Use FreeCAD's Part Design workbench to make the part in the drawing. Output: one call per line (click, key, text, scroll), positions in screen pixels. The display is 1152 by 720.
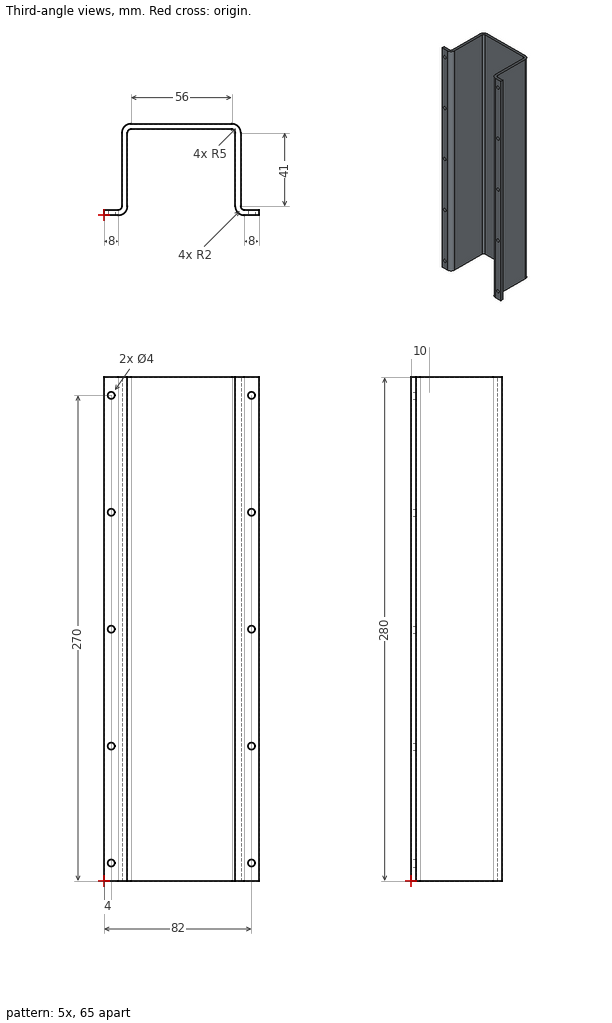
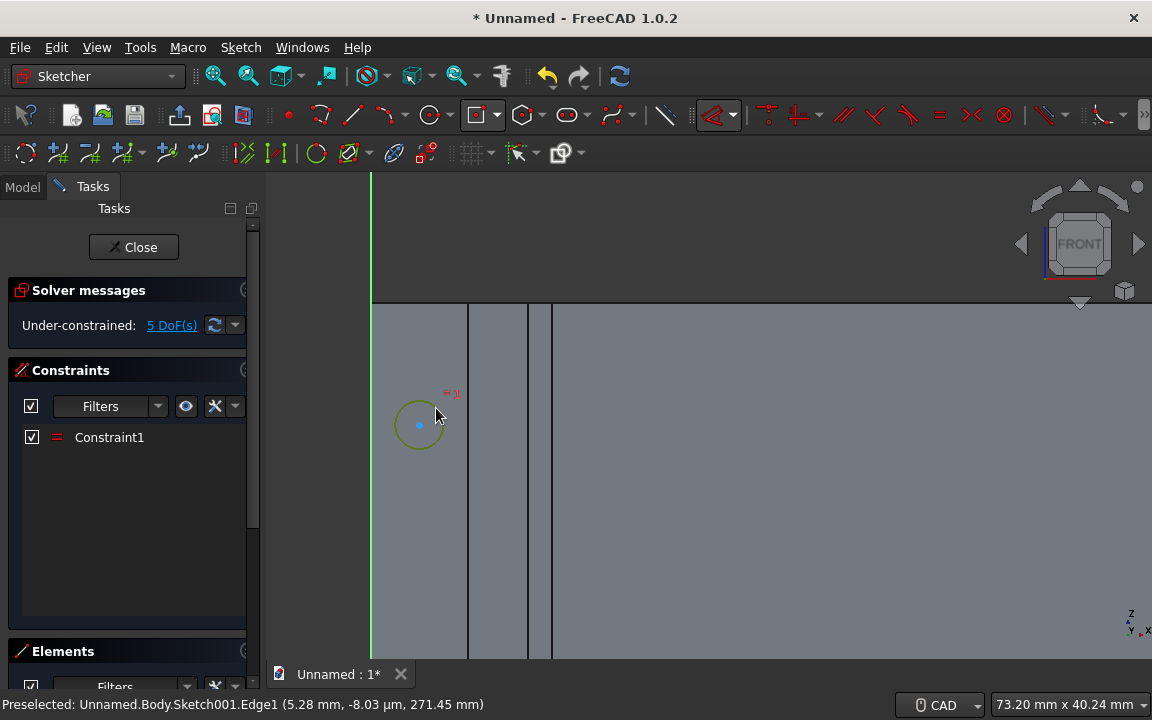
key(k)
key(o)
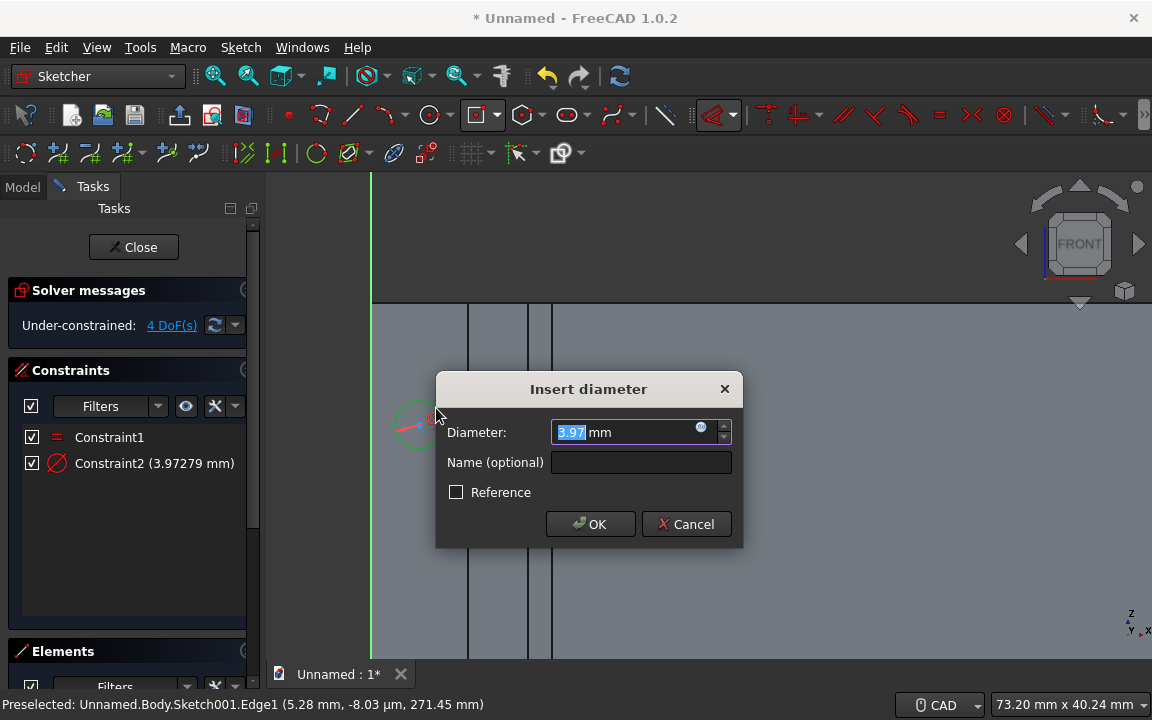
text(4)
key(Return)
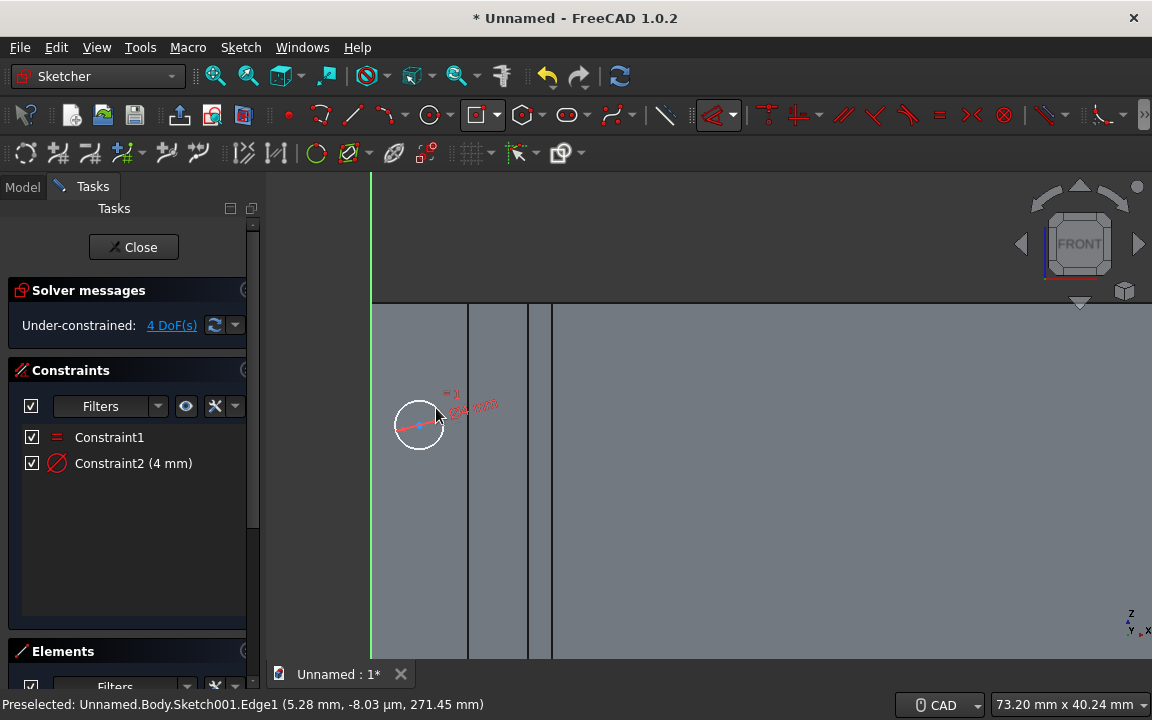
click(419, 425)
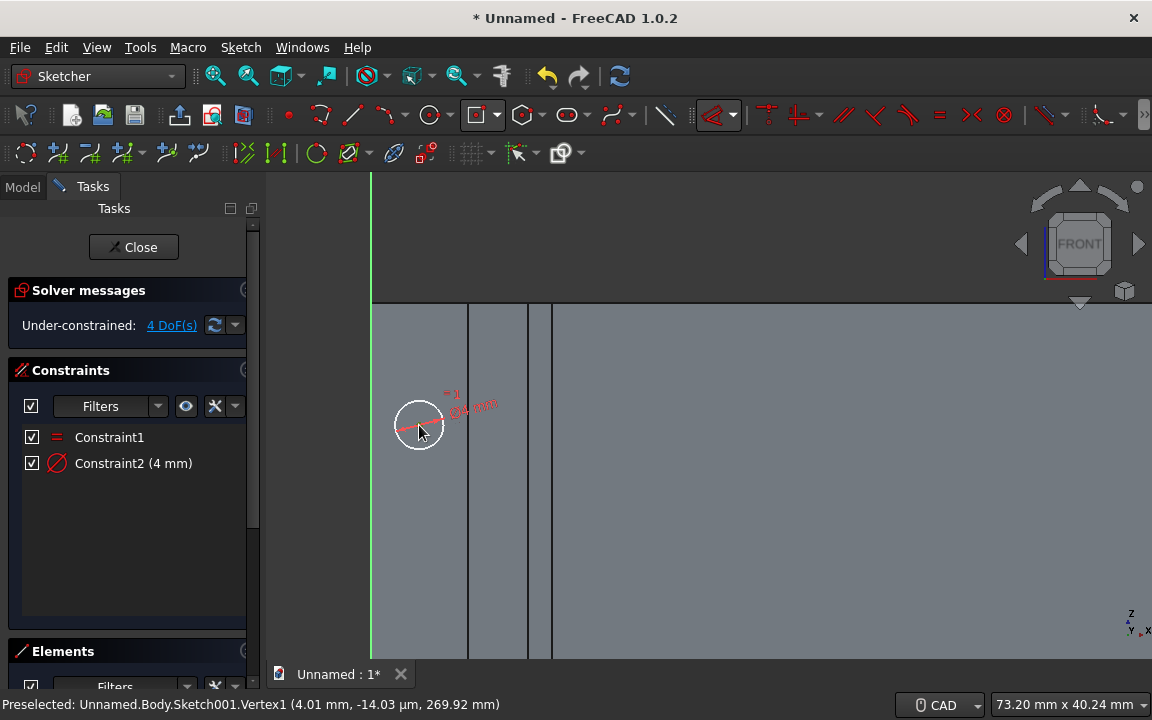
key(l)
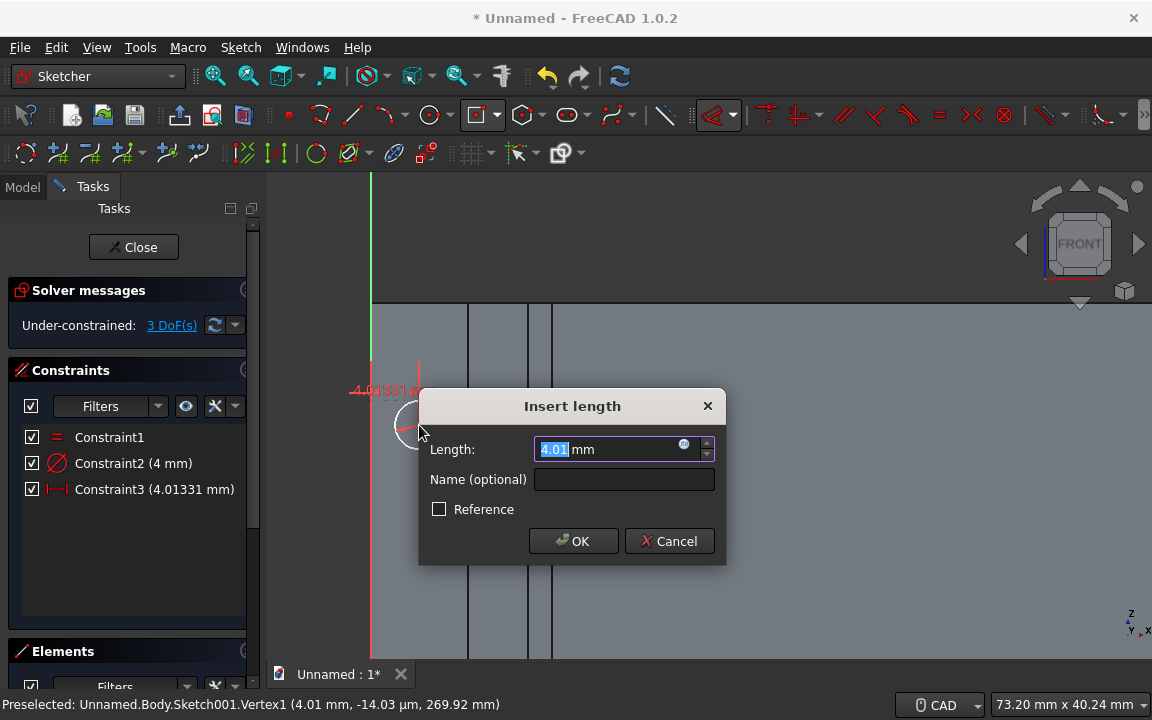
text(4)
key(Return)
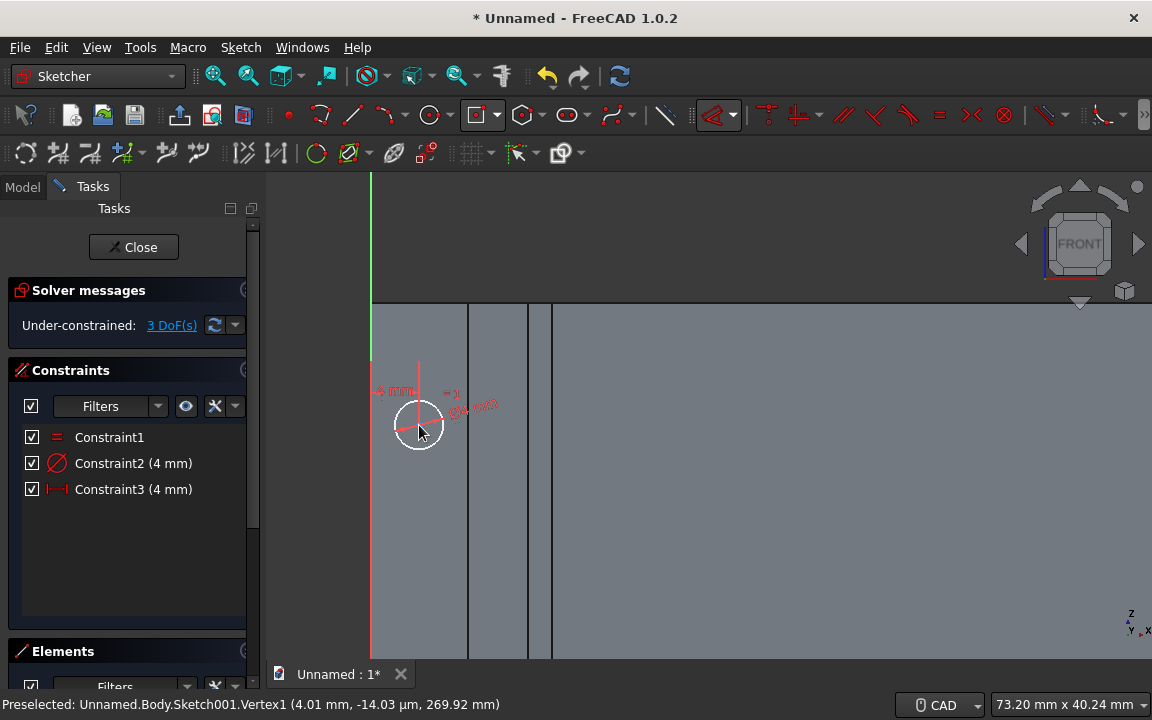
scroll(436, 408, down, 4)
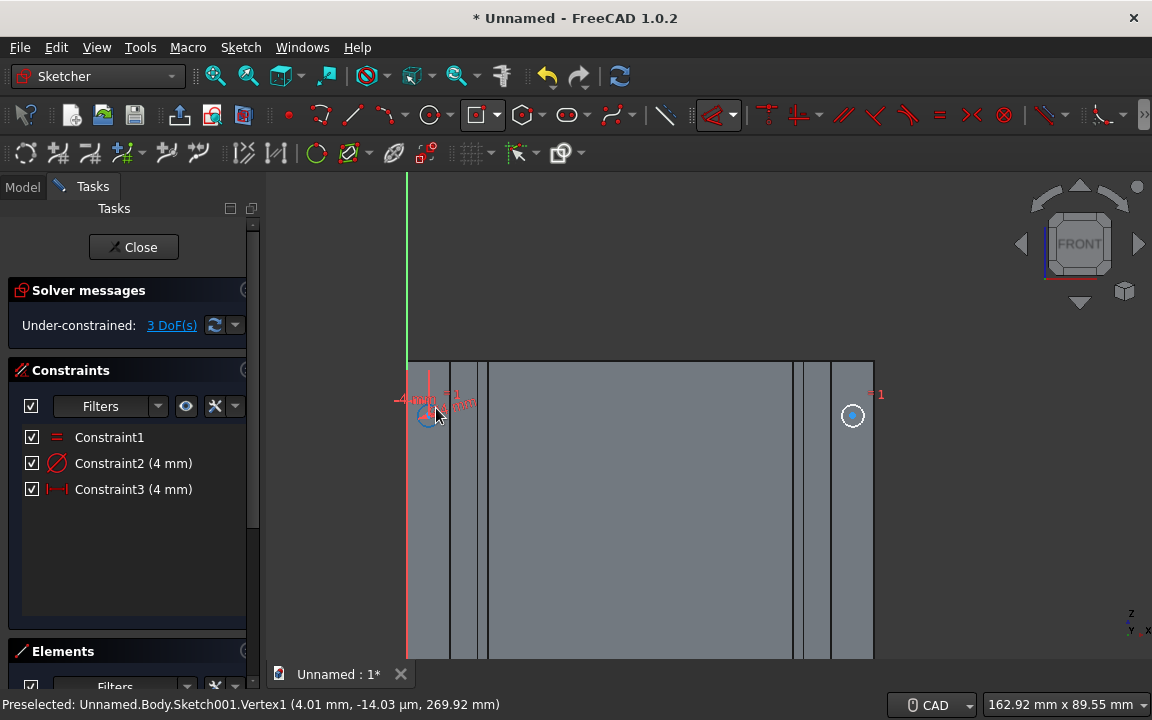
click(853, 416)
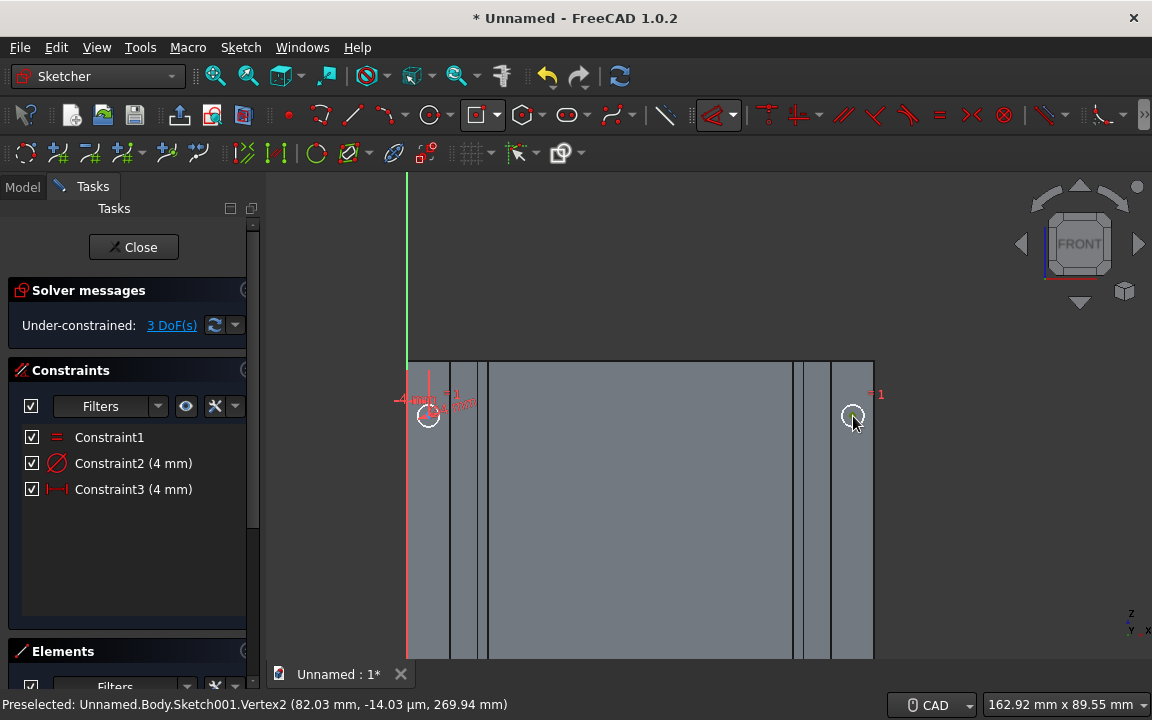
key(l)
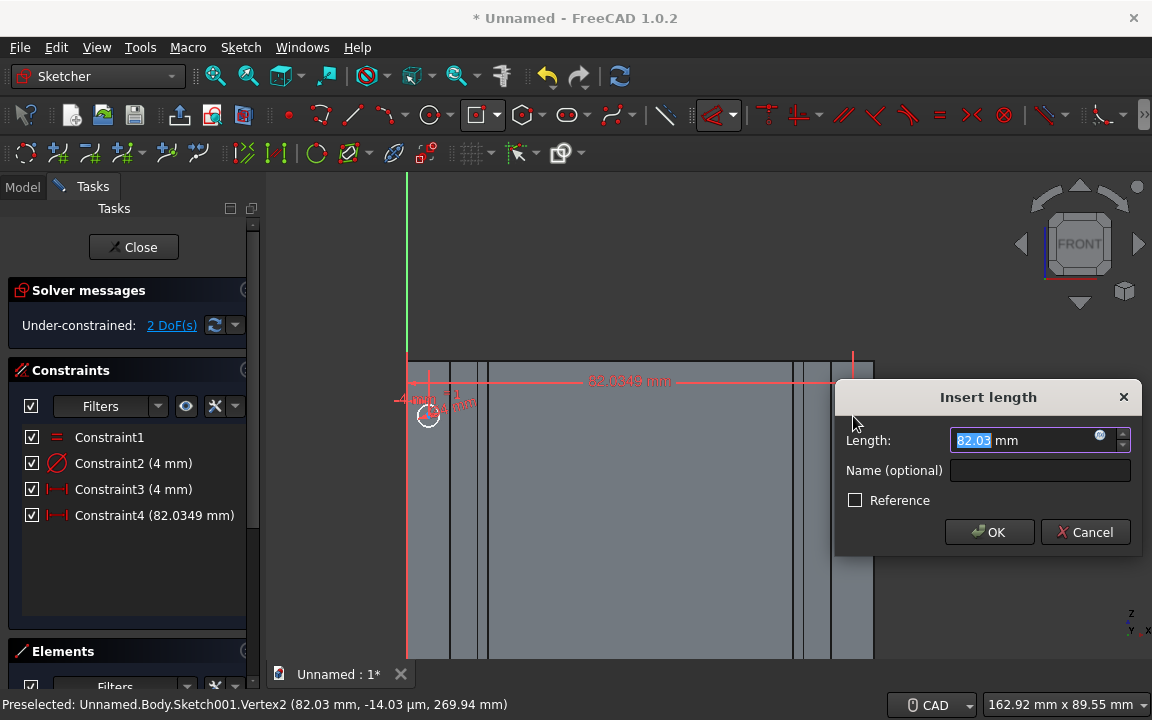
text(82)
key(Return)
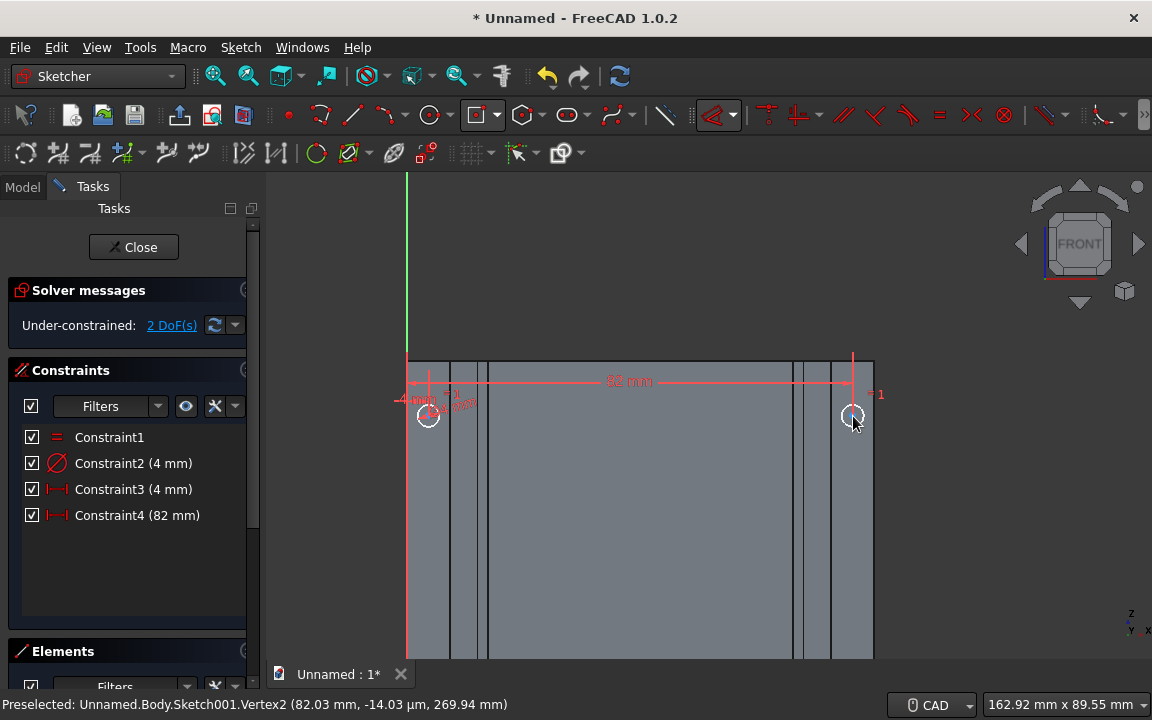
click(429, 416)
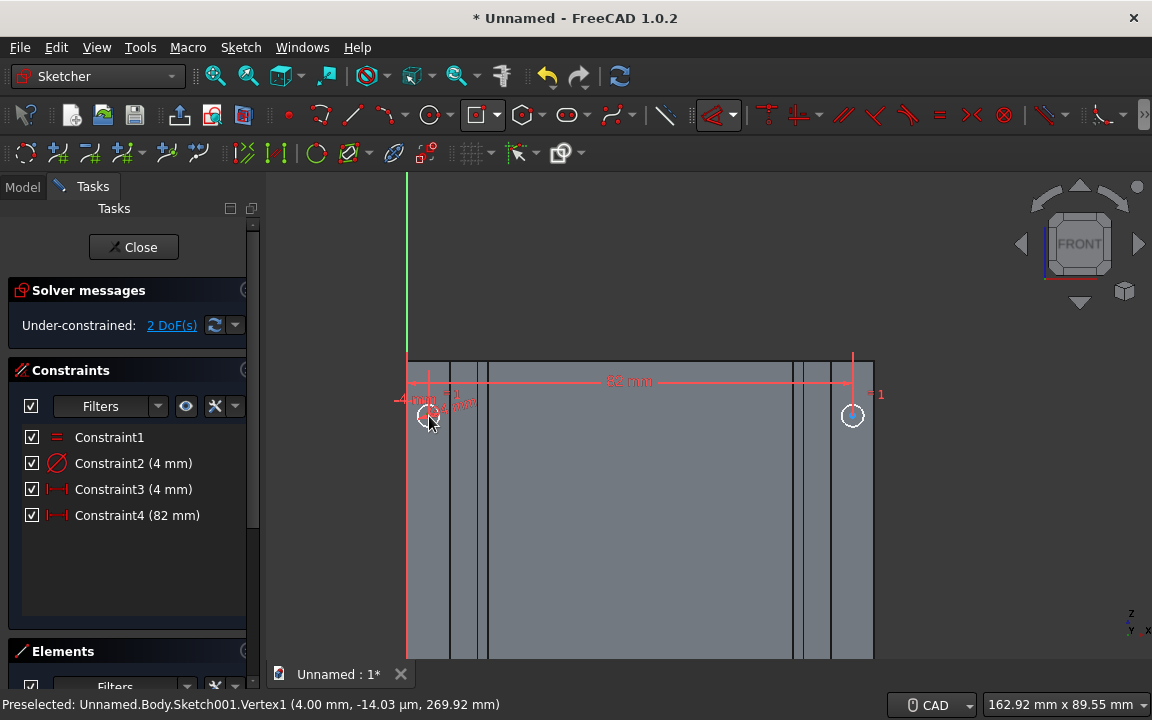
key(i)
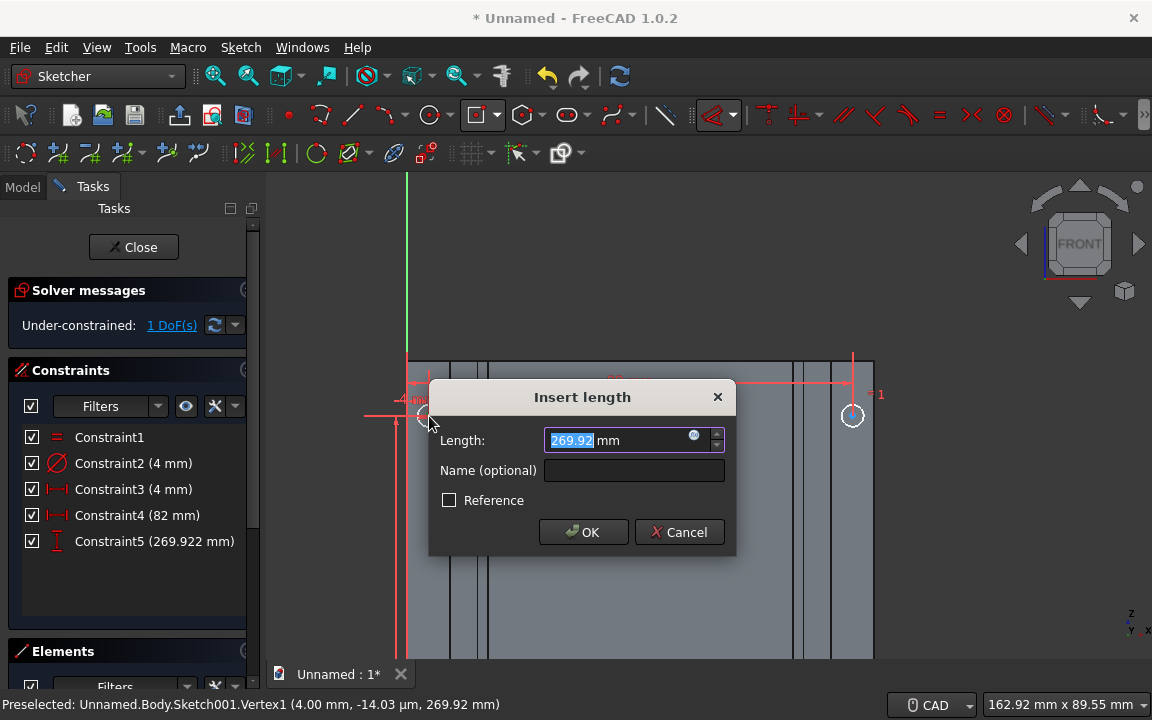
text(270)
key(Return)